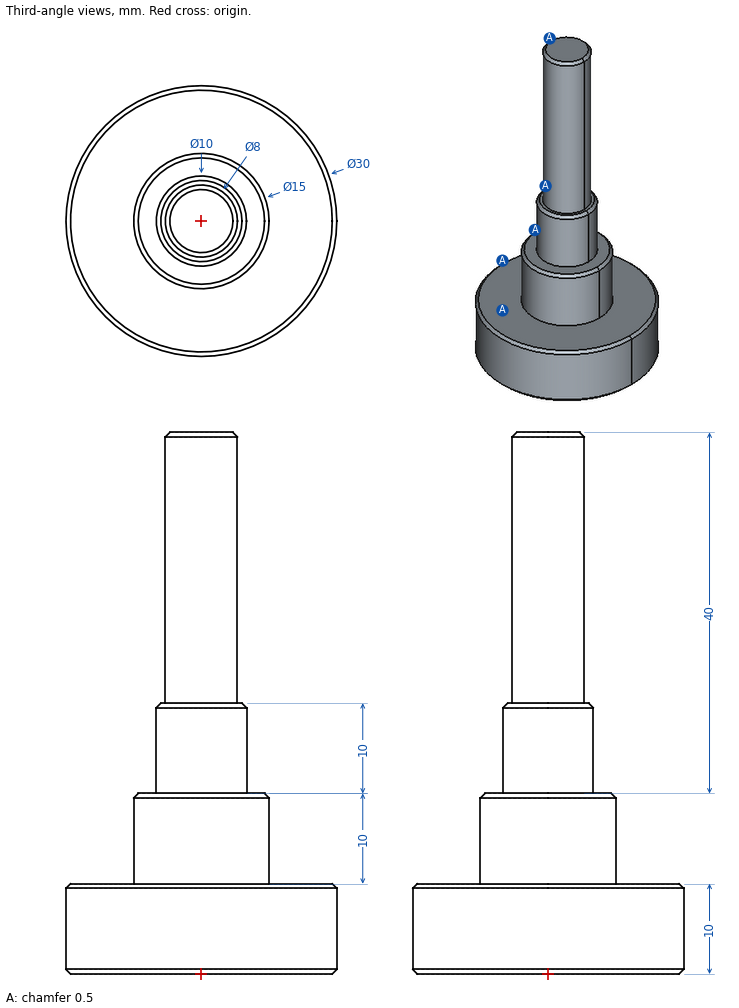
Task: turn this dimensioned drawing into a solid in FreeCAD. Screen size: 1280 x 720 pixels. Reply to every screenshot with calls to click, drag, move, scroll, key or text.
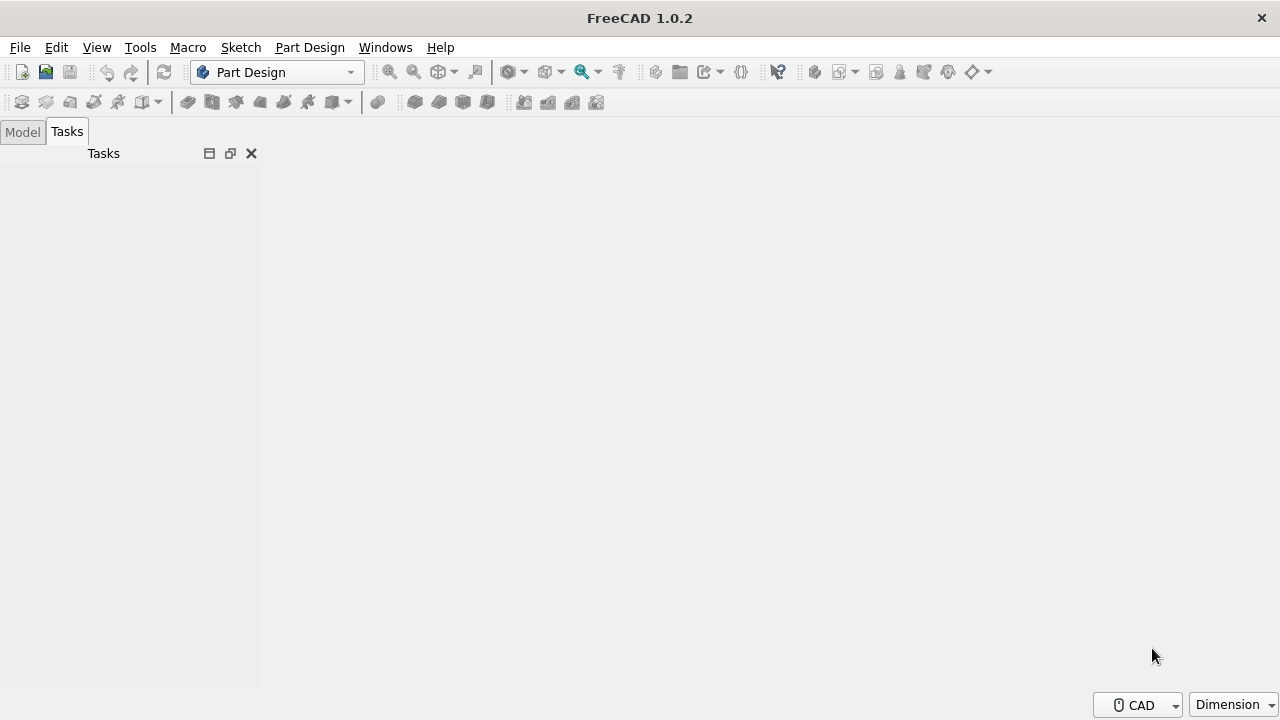
click(22, 72)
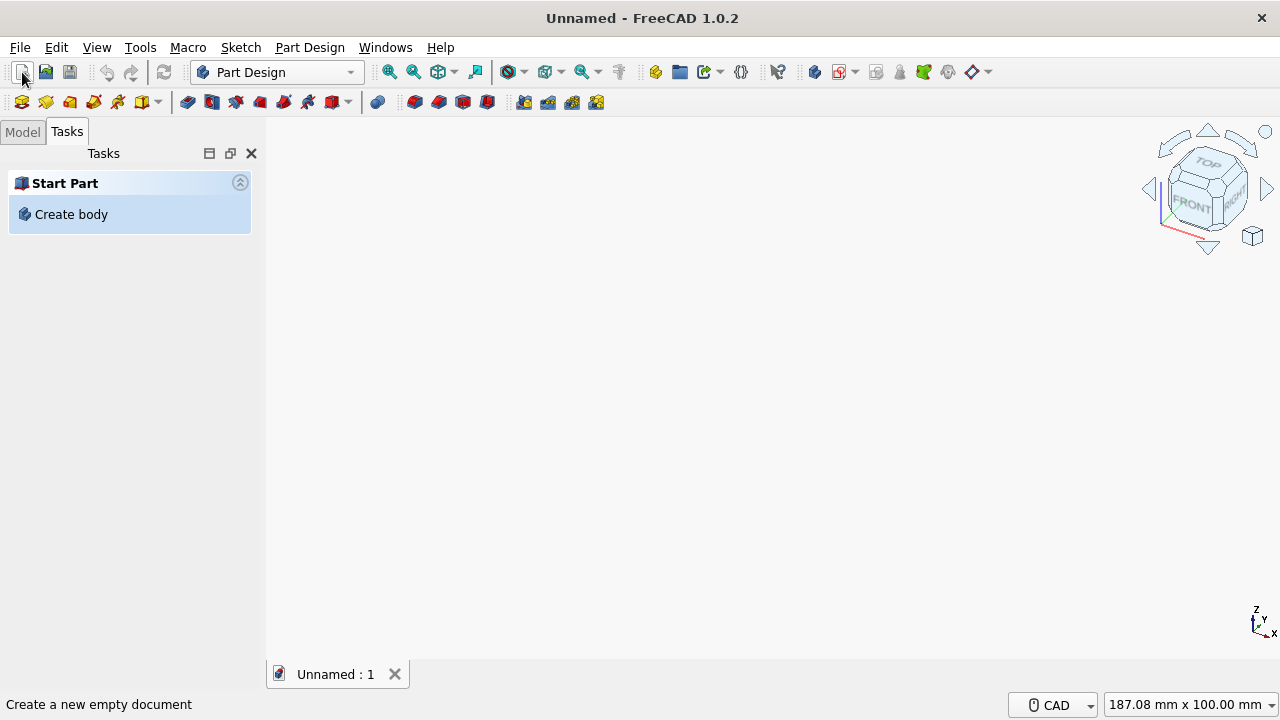
click(840, 72)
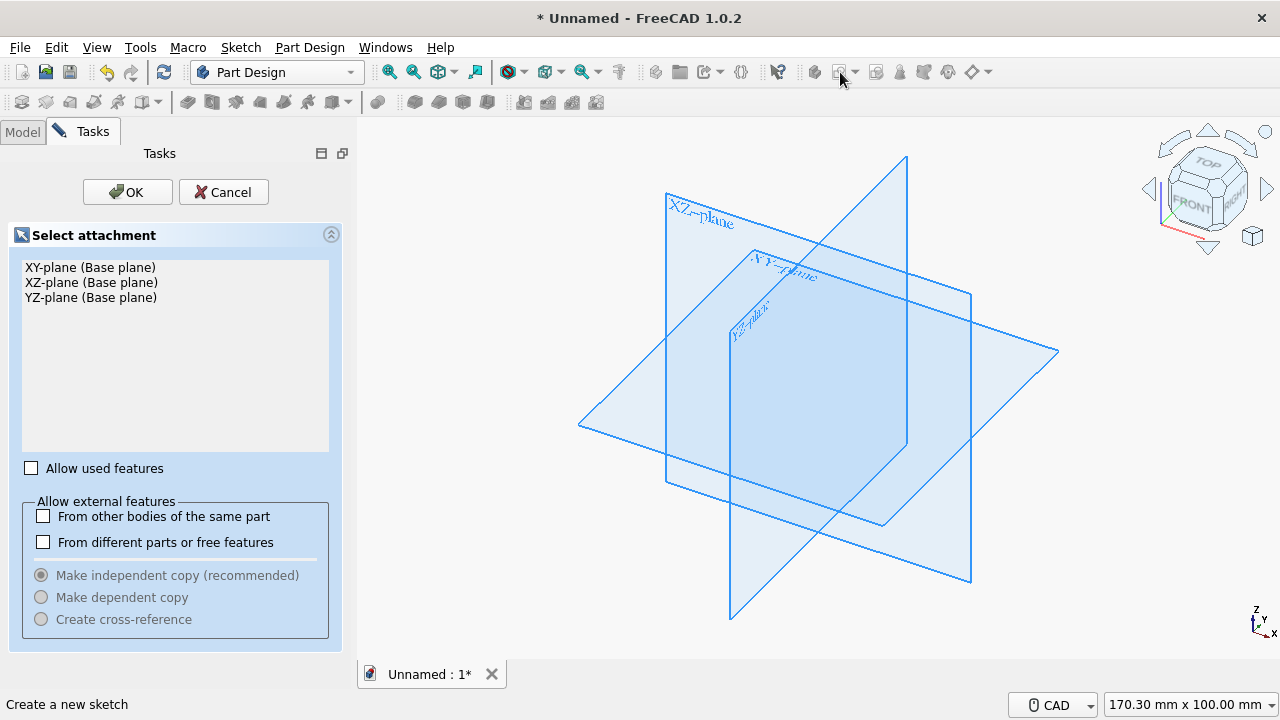
click(82, 268)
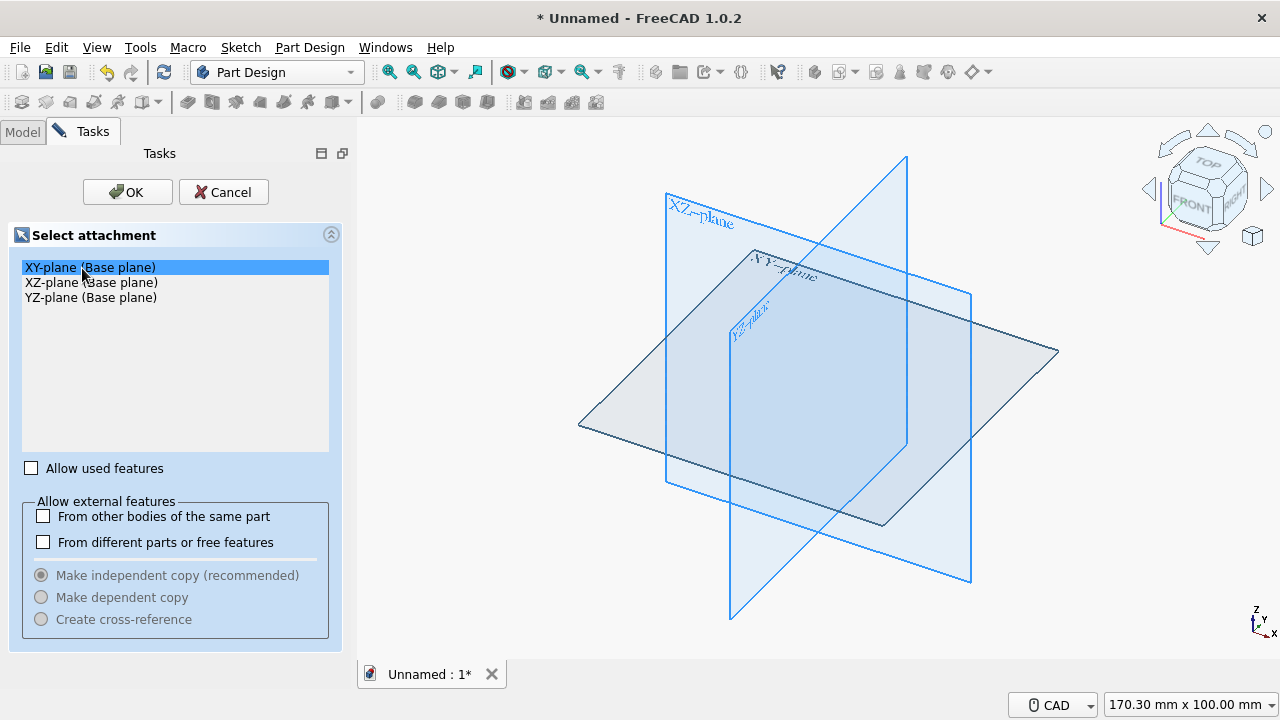
click(128, 192)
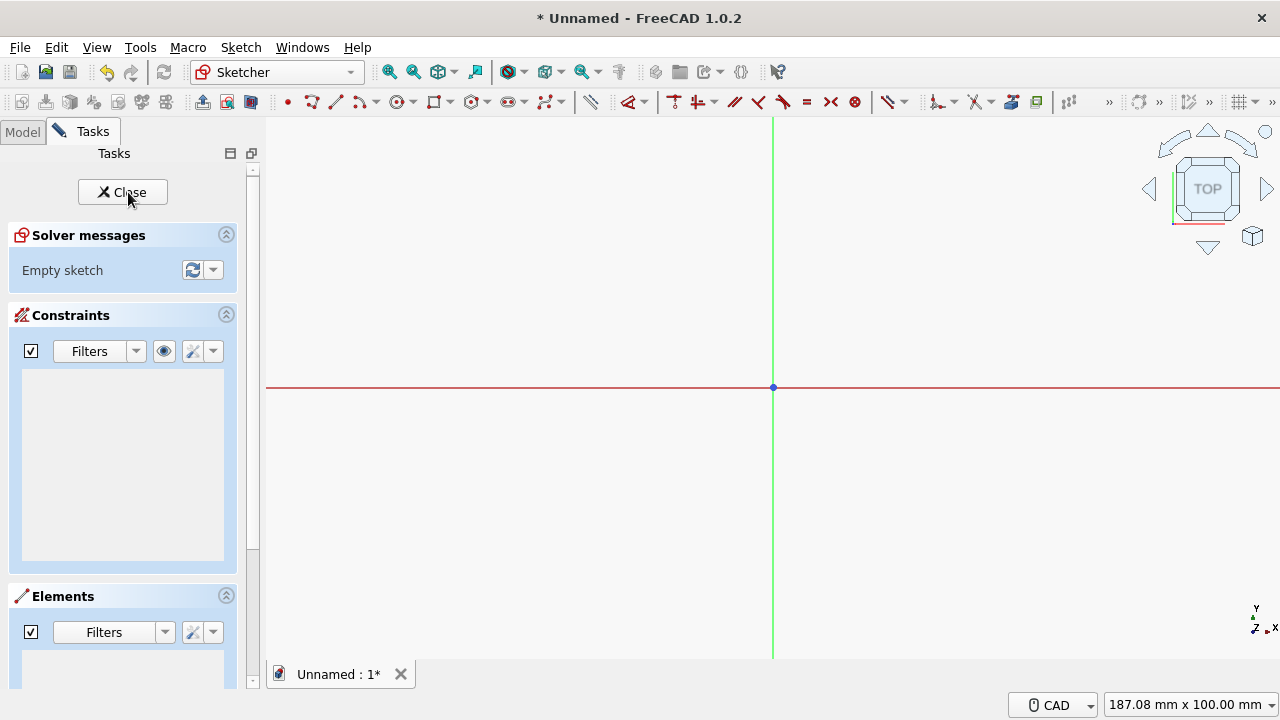
scroll(829, 388, up, 4)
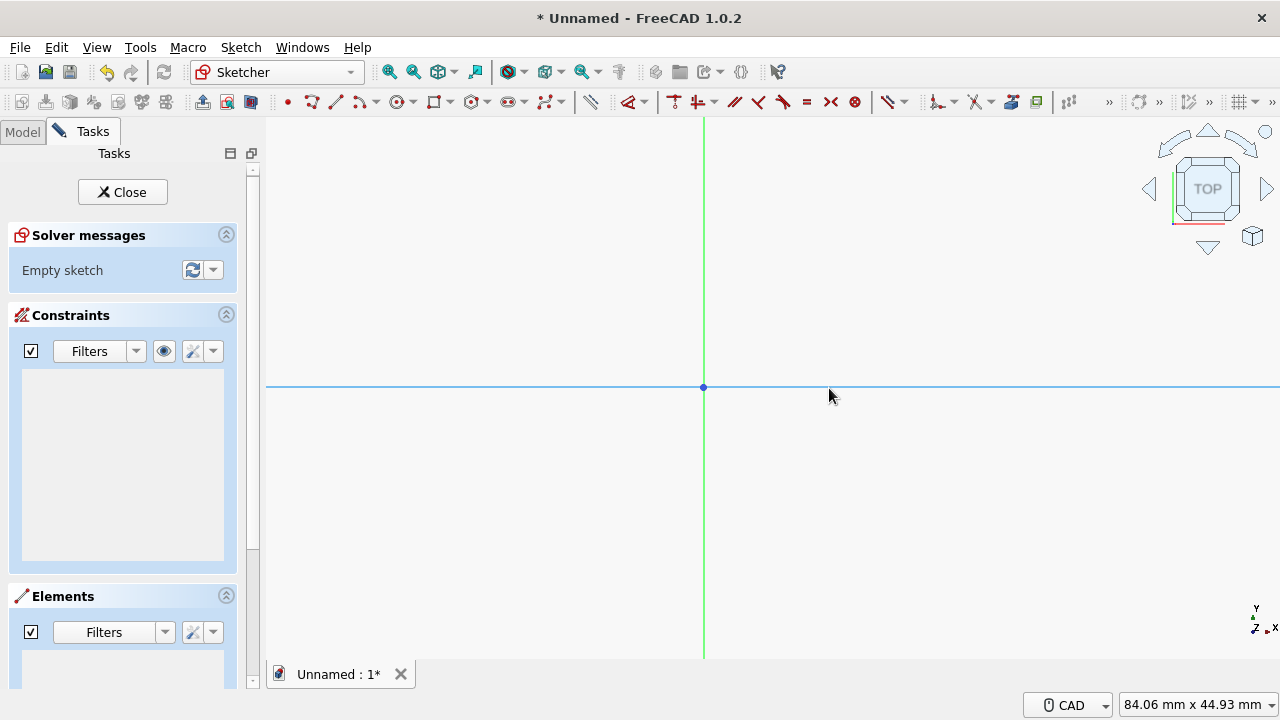
click(398, 102)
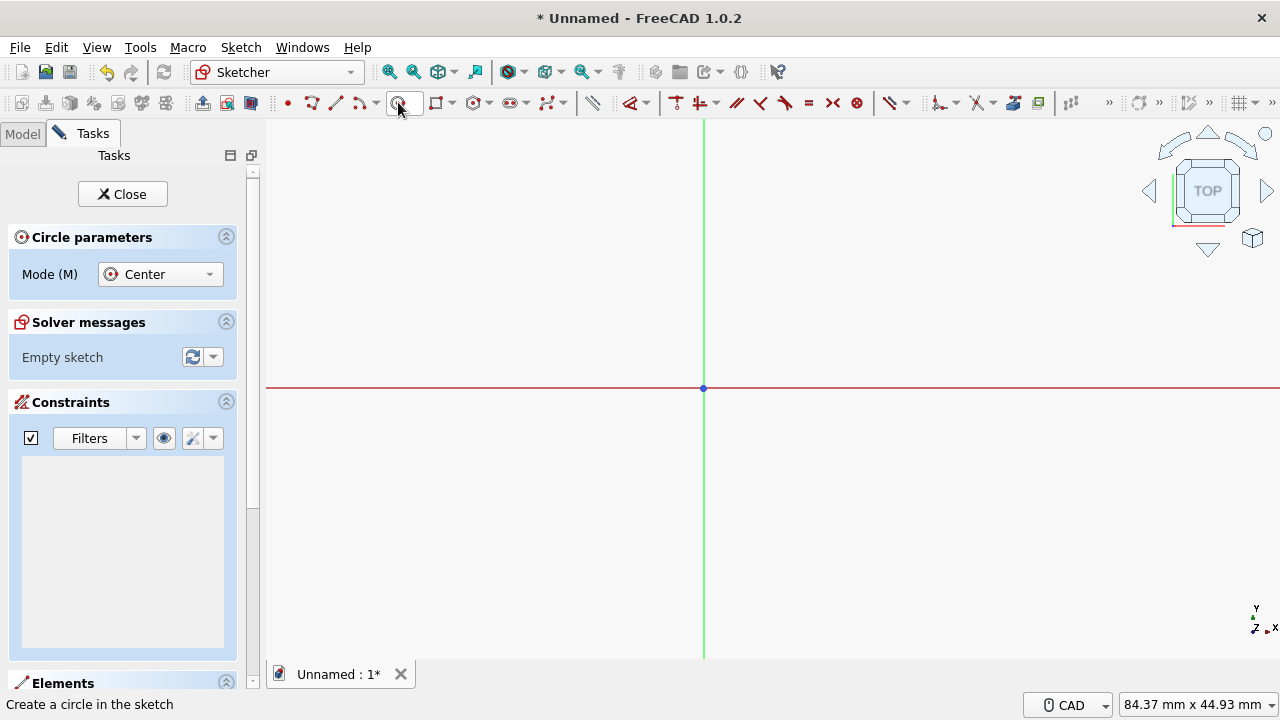
click(704, 388)
click(831, 261)
key(Escape)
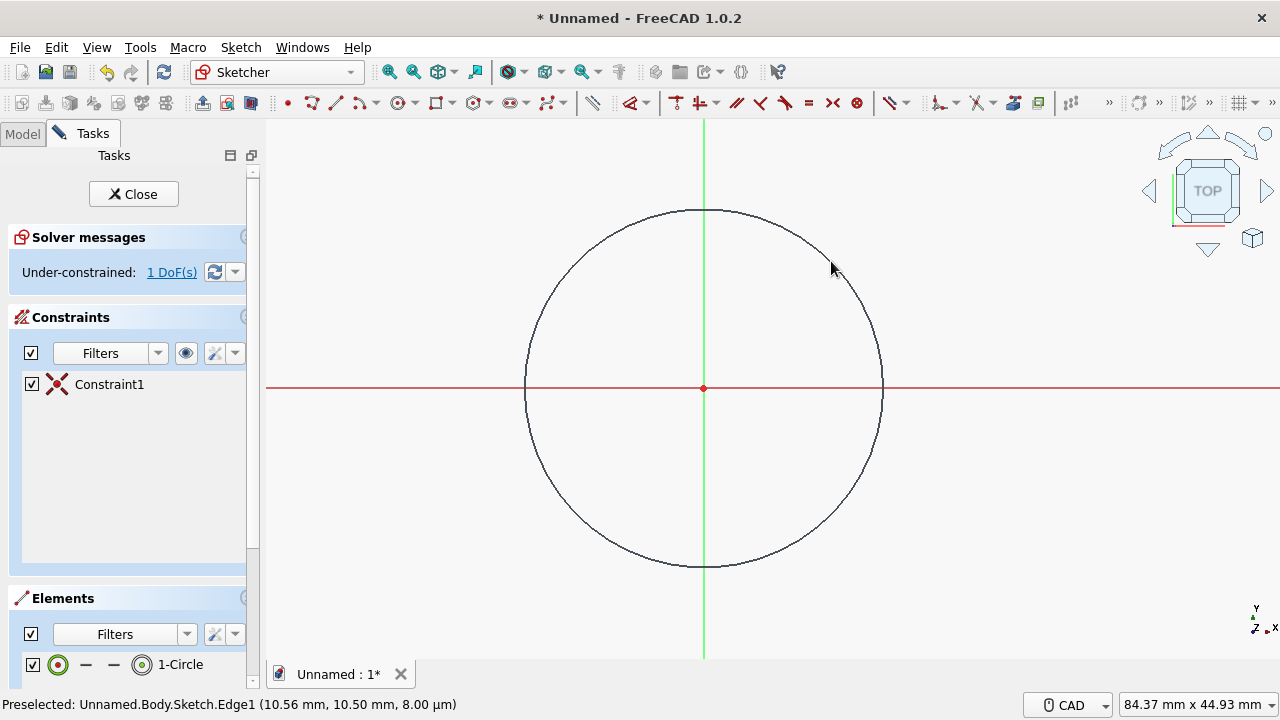
click(830, 261)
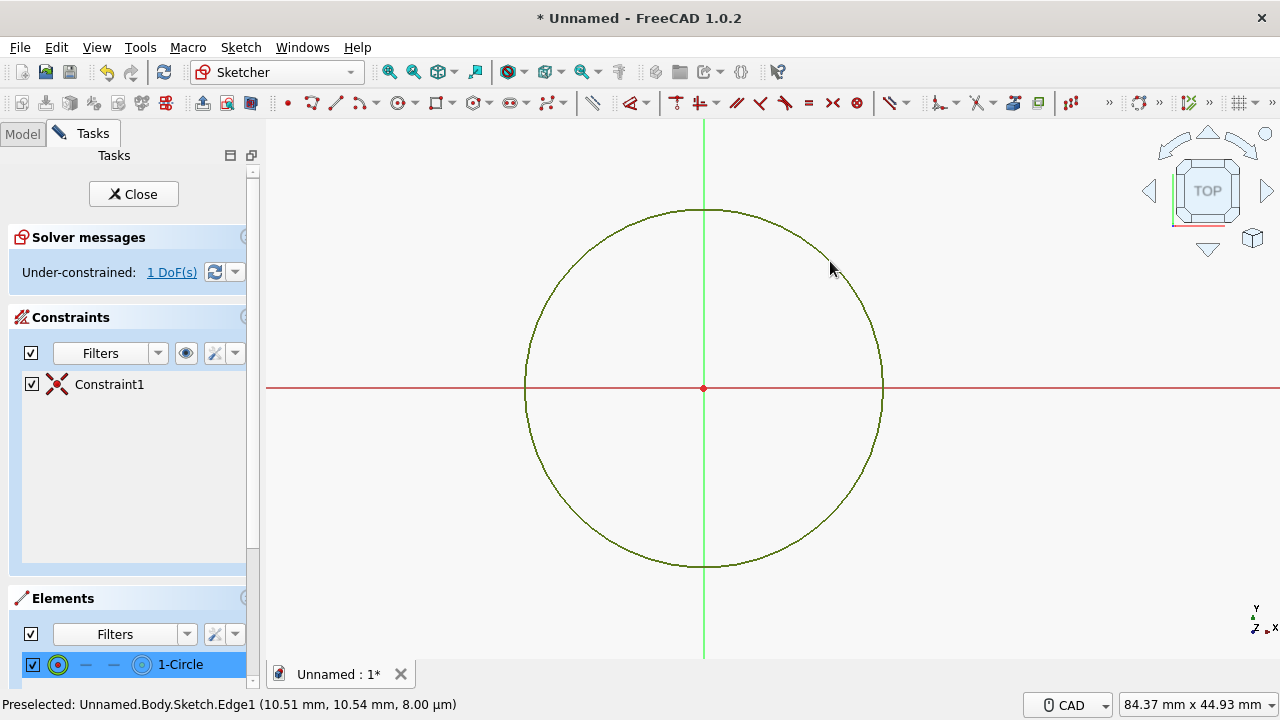
key(k)
key(o)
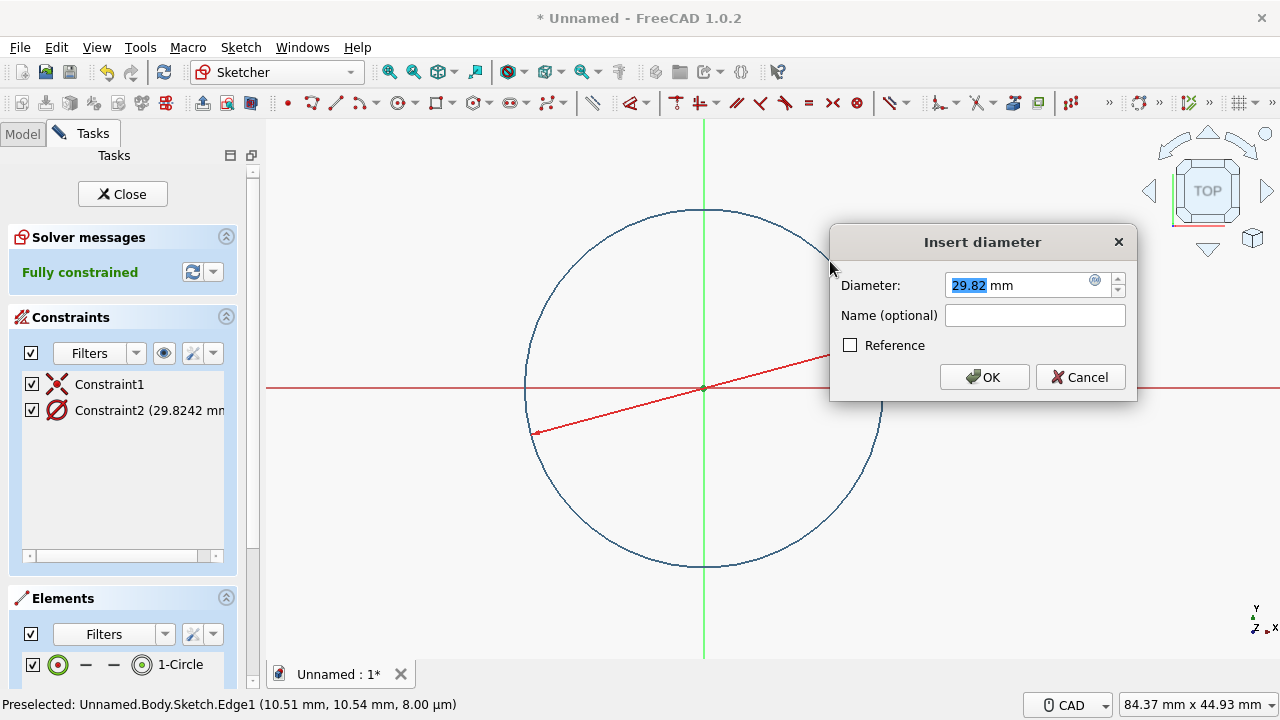
text(30)
key(Return)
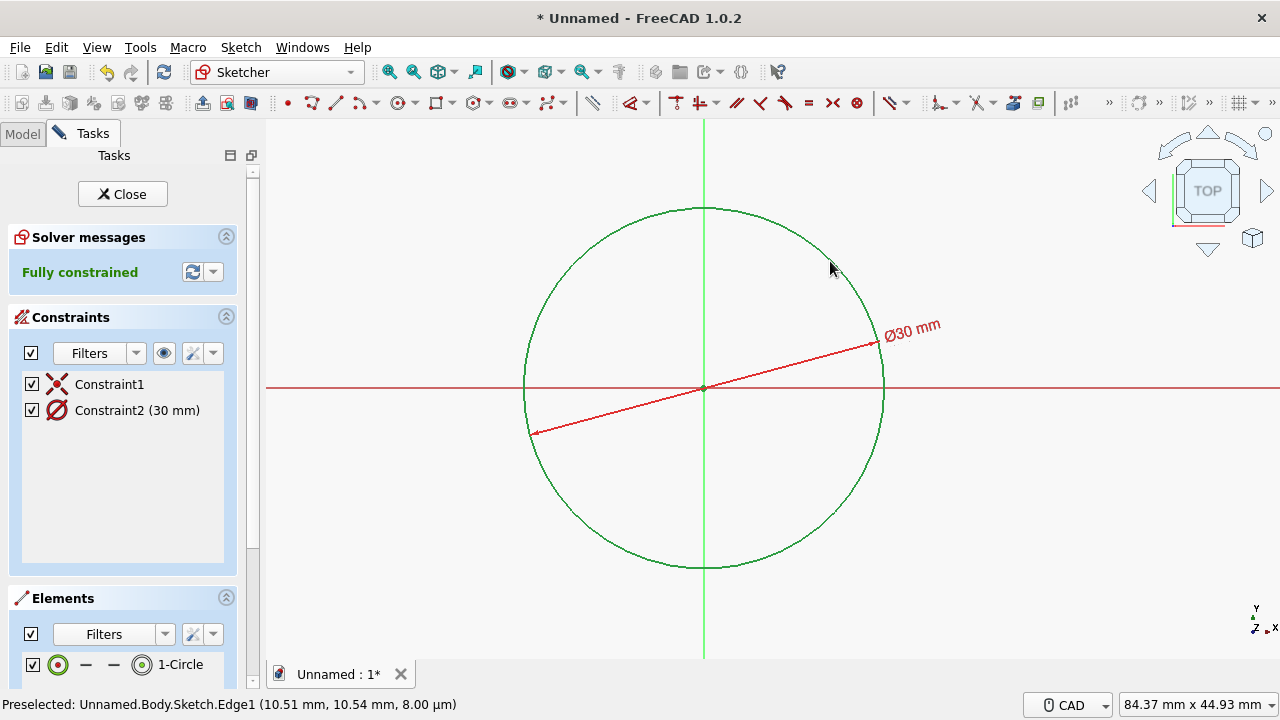
click(123, 194)